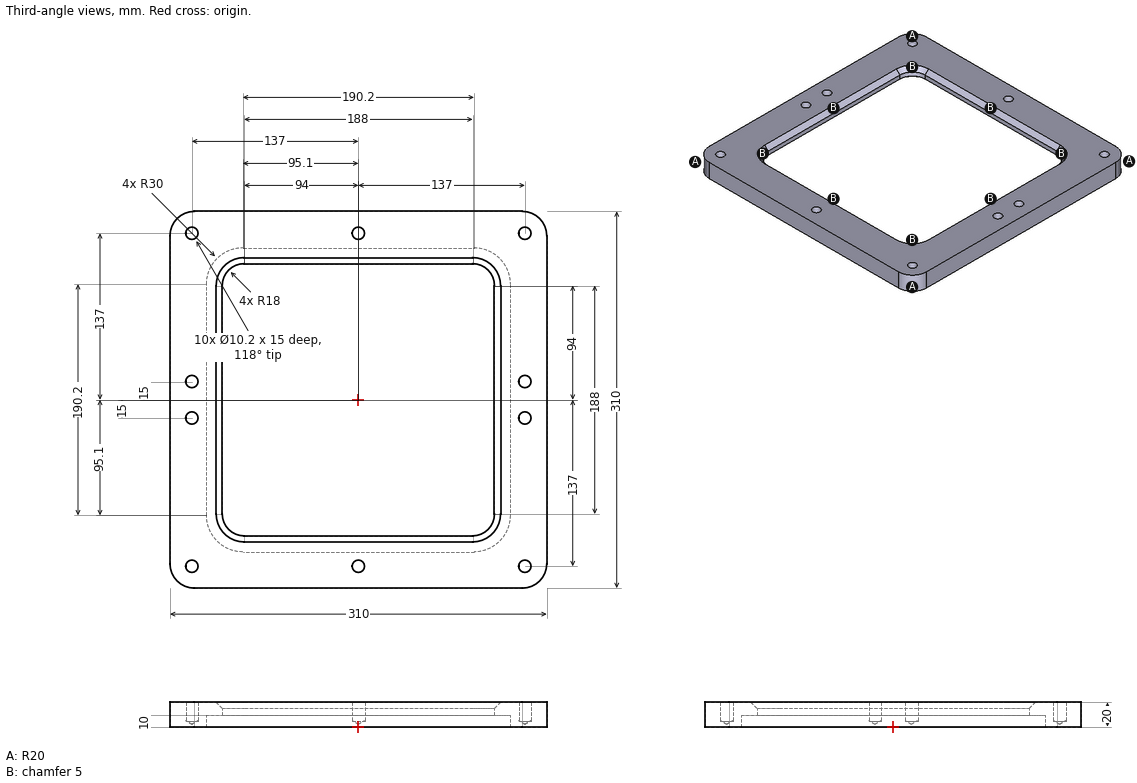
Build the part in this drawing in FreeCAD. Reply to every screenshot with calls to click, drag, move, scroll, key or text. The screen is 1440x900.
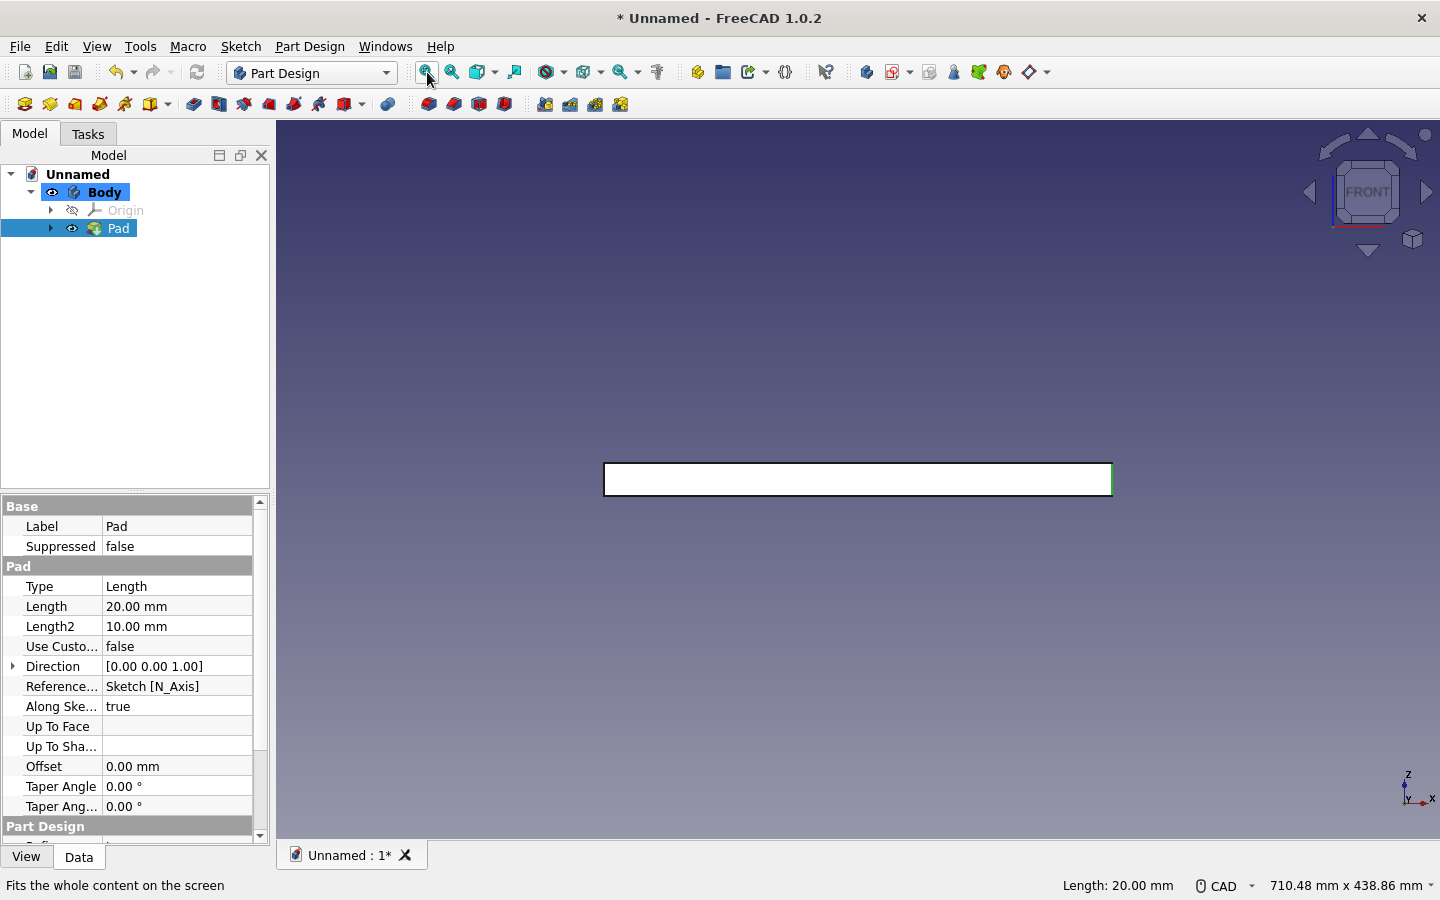
click(604, 479, ctrl)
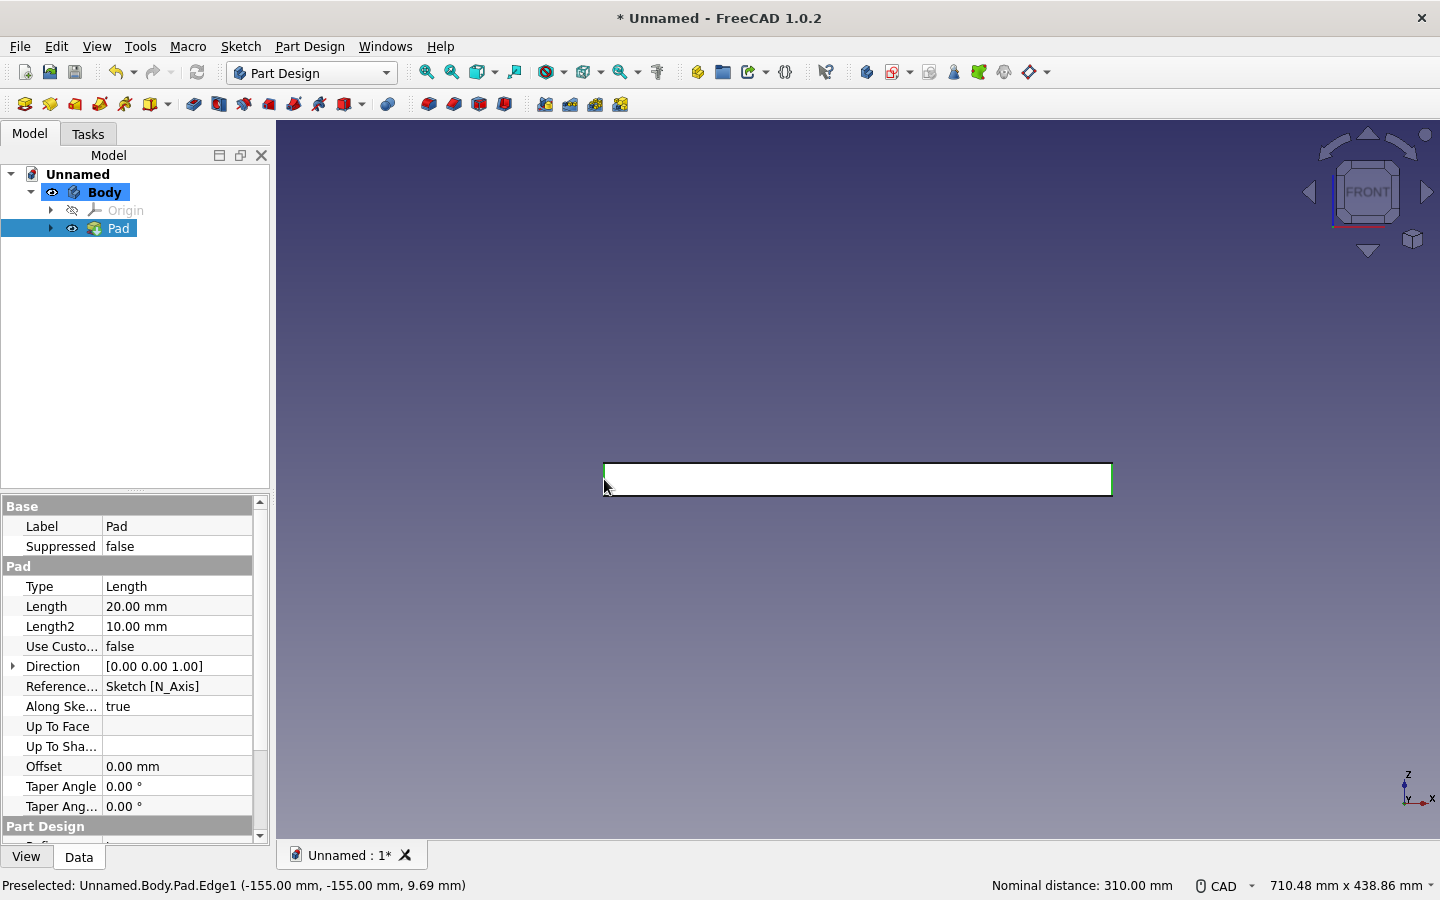
key(3)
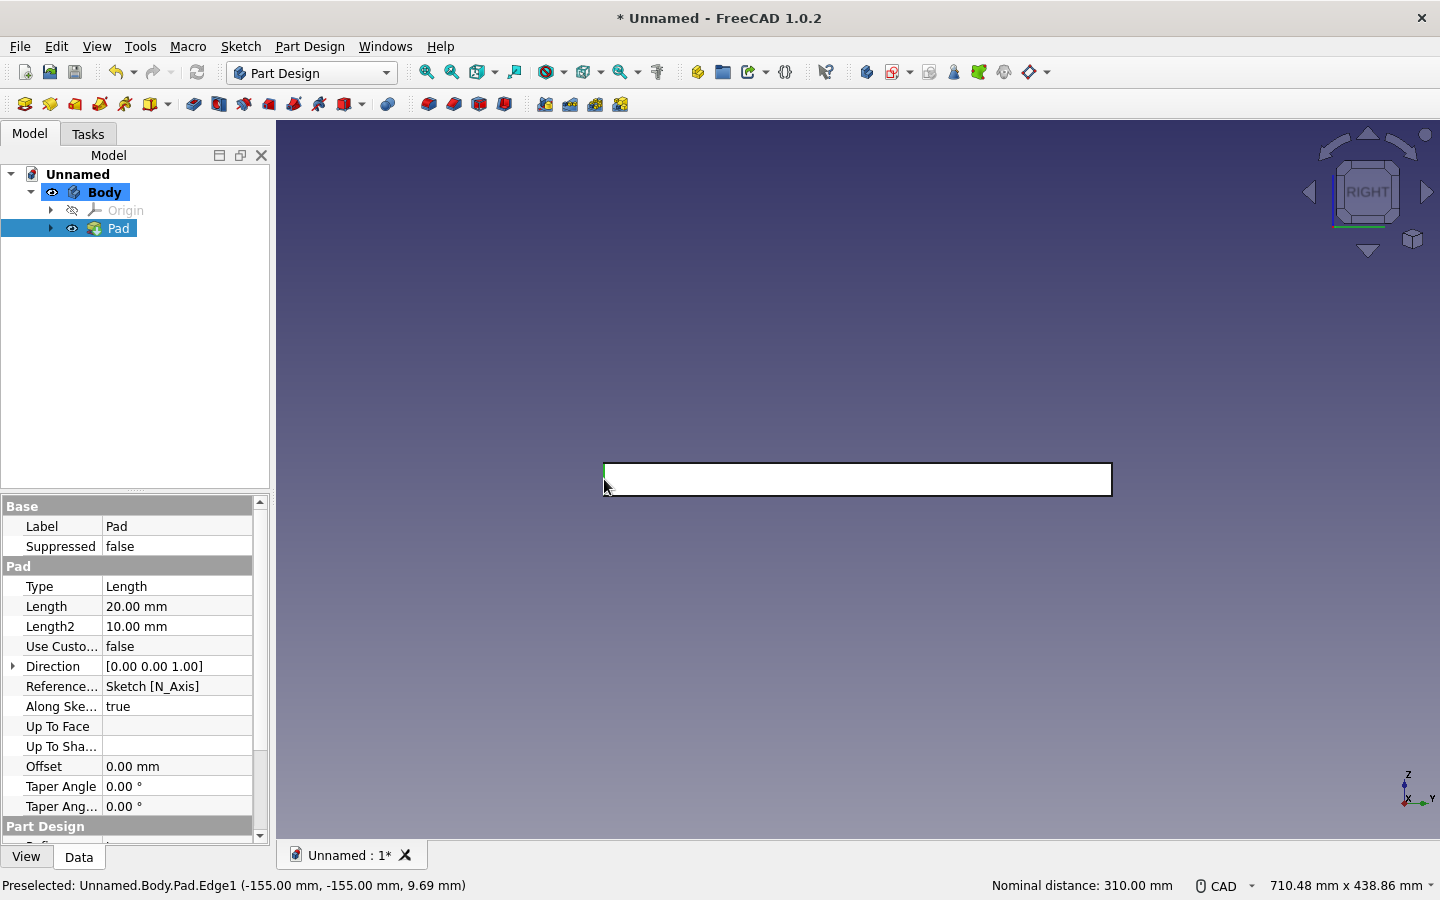
click(427, 72)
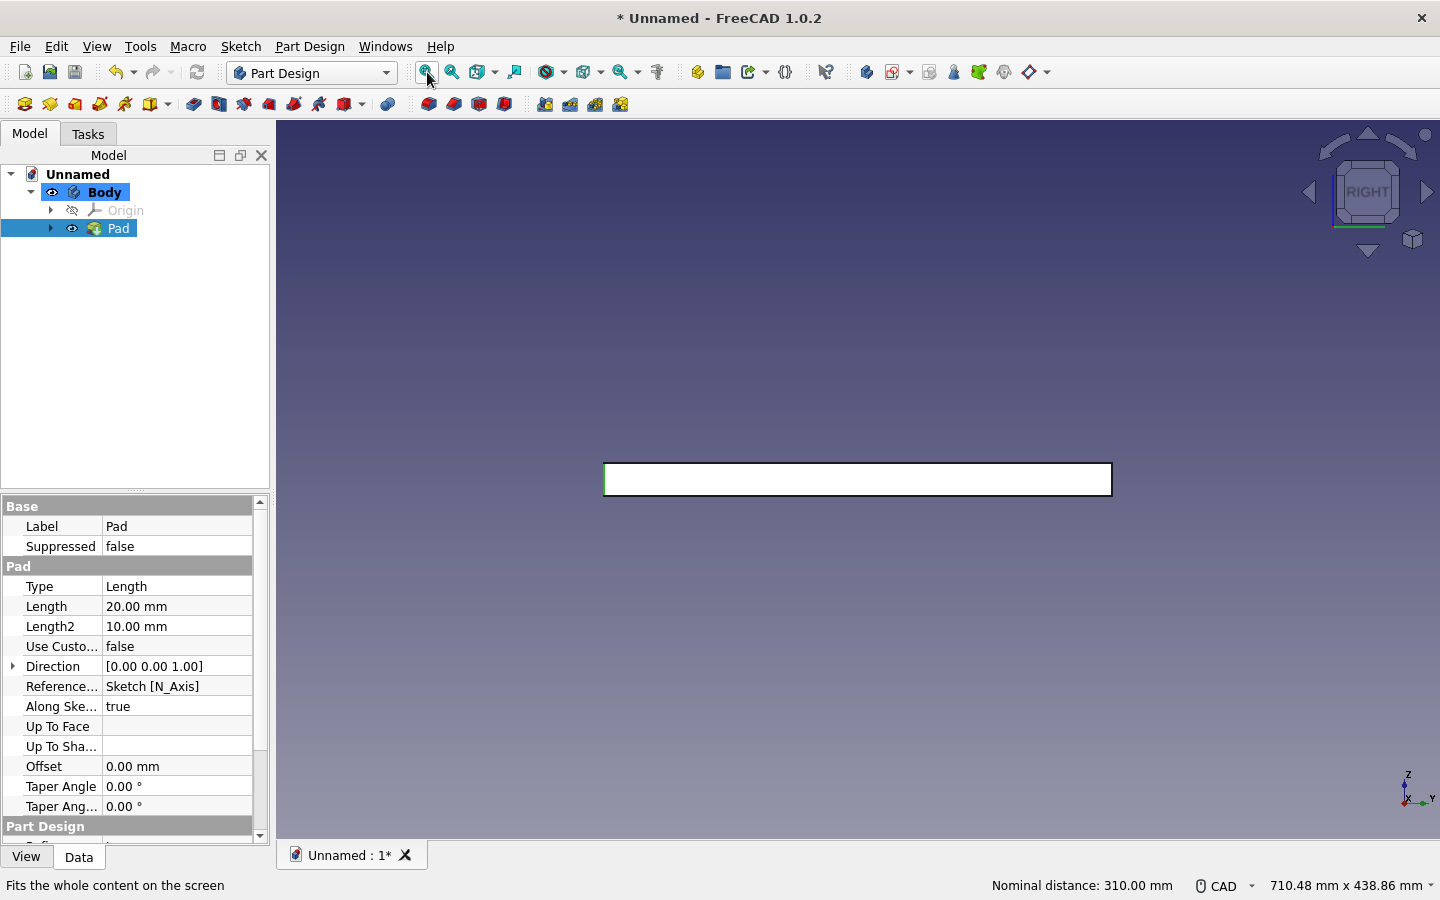
click(1112, 478, ctrl)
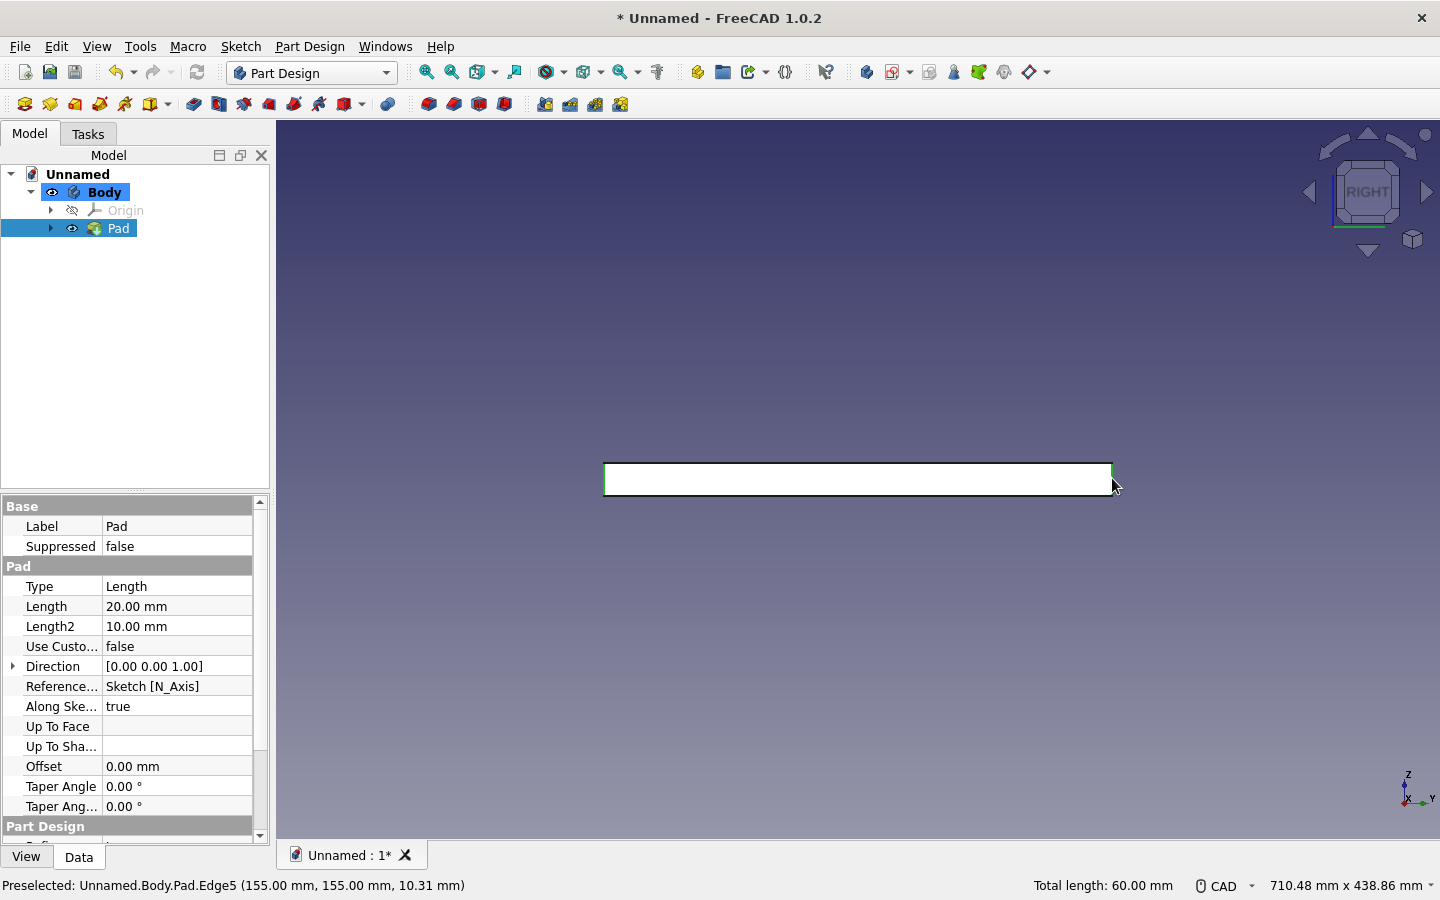
key(5)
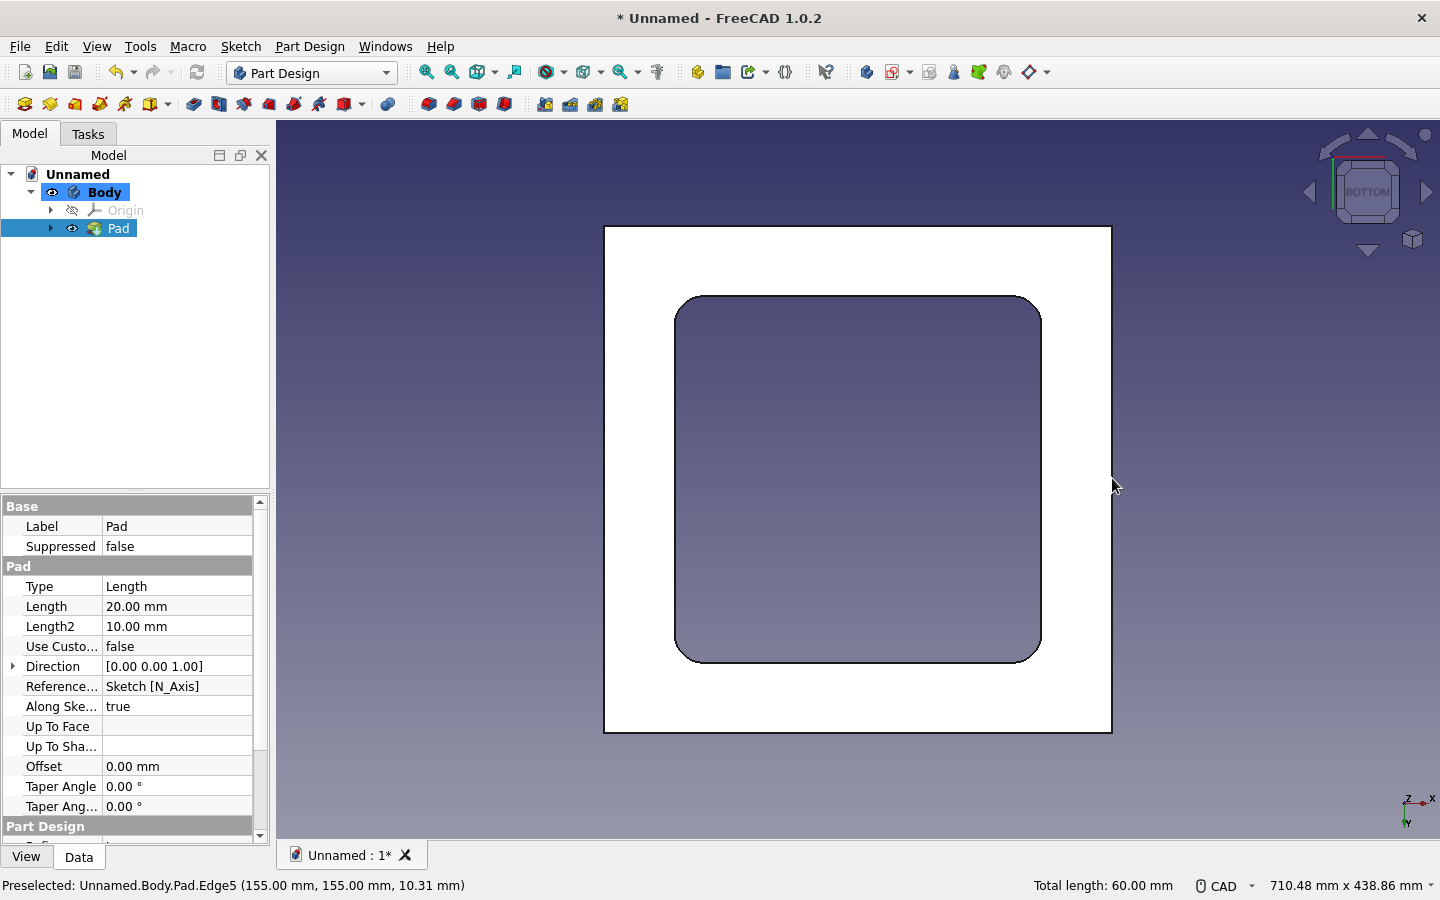
key(4)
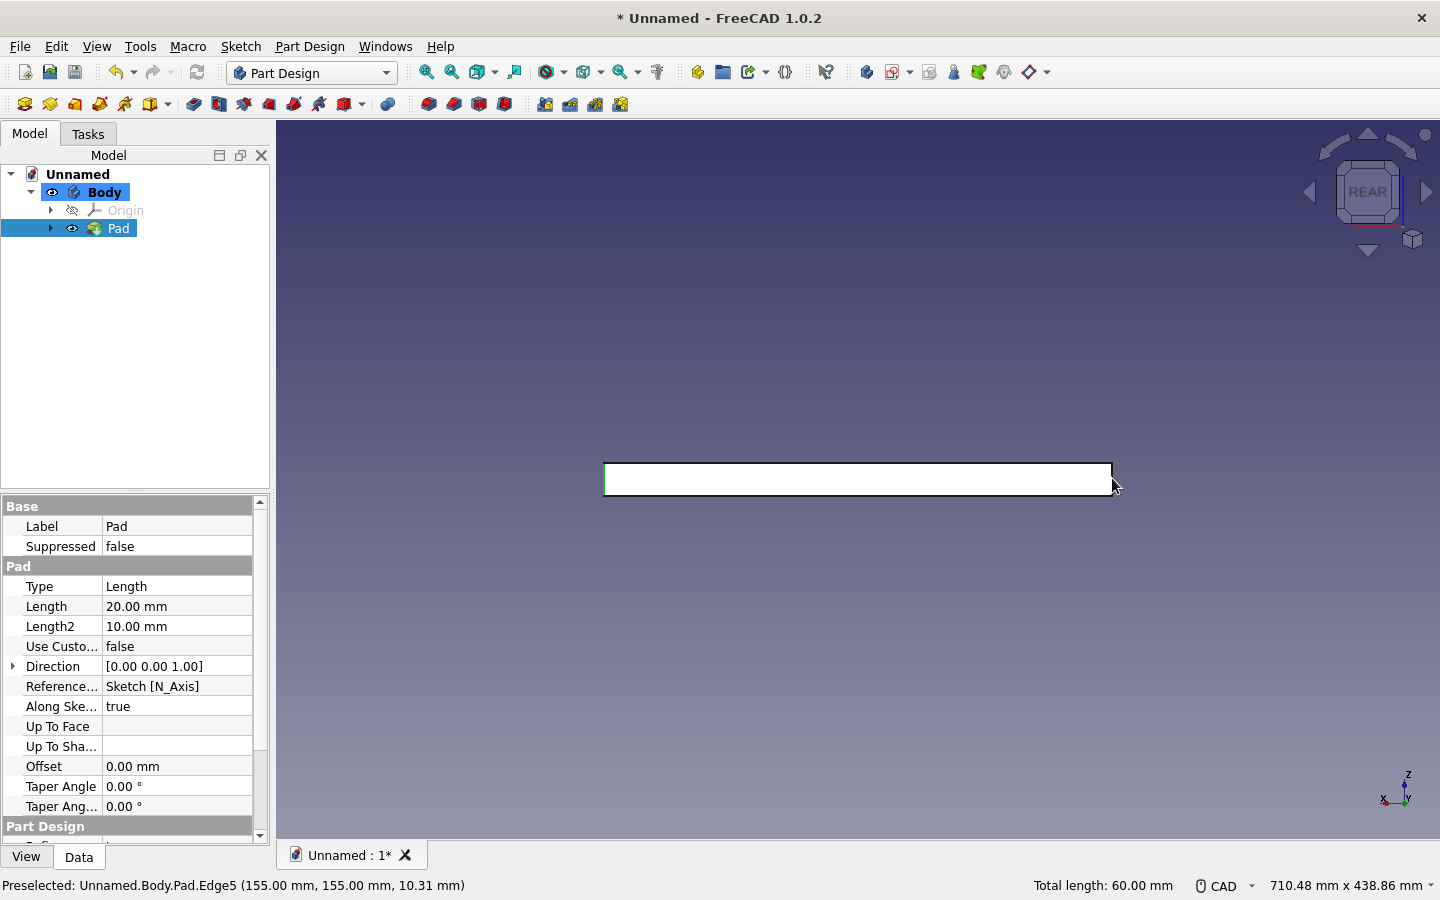
click(427, 72)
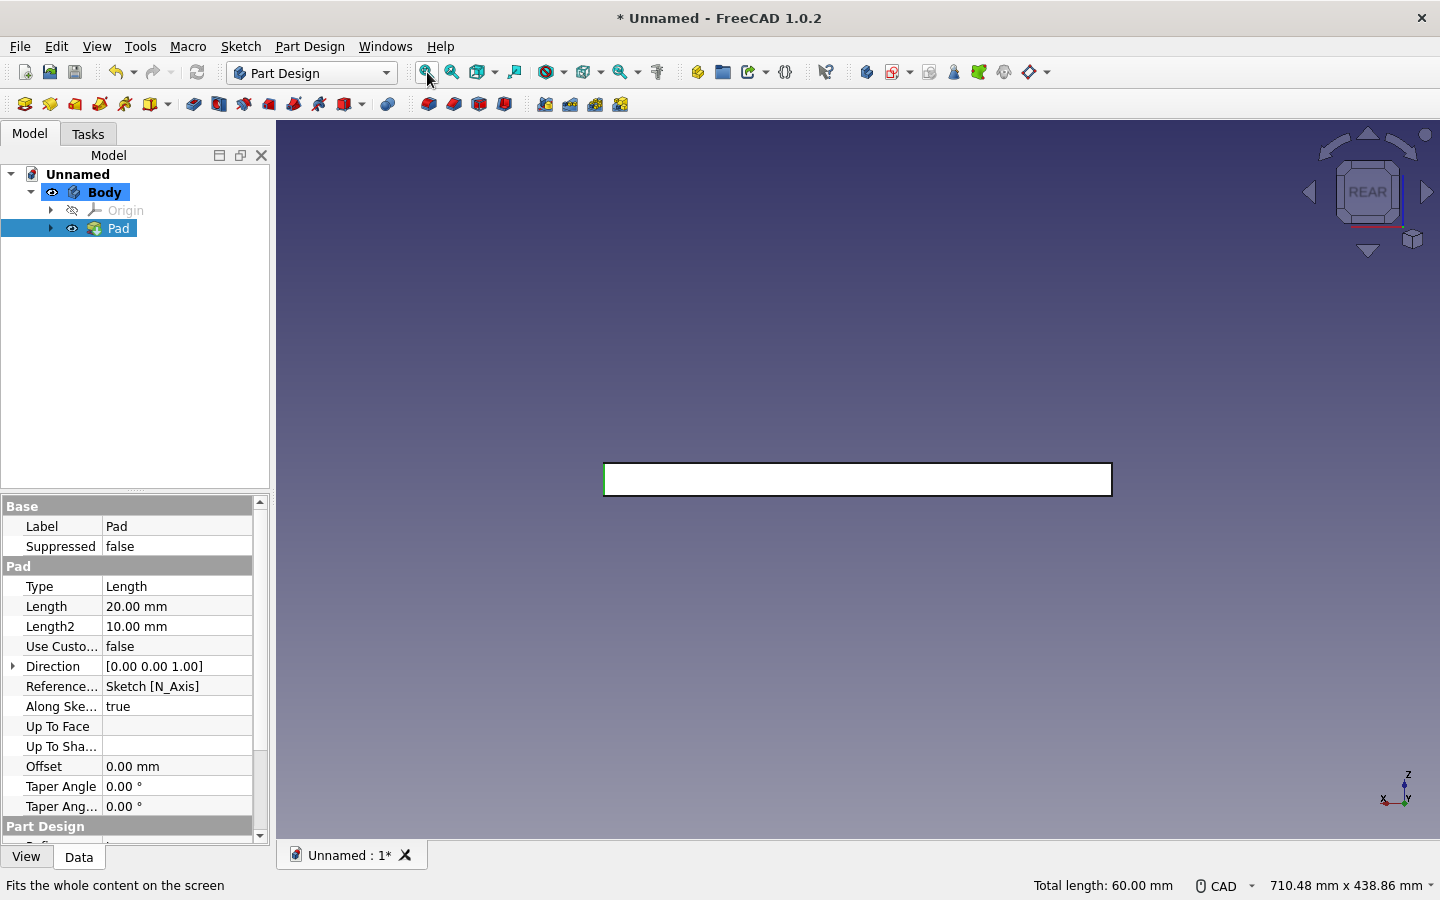
click(1112, 479, ctrl)